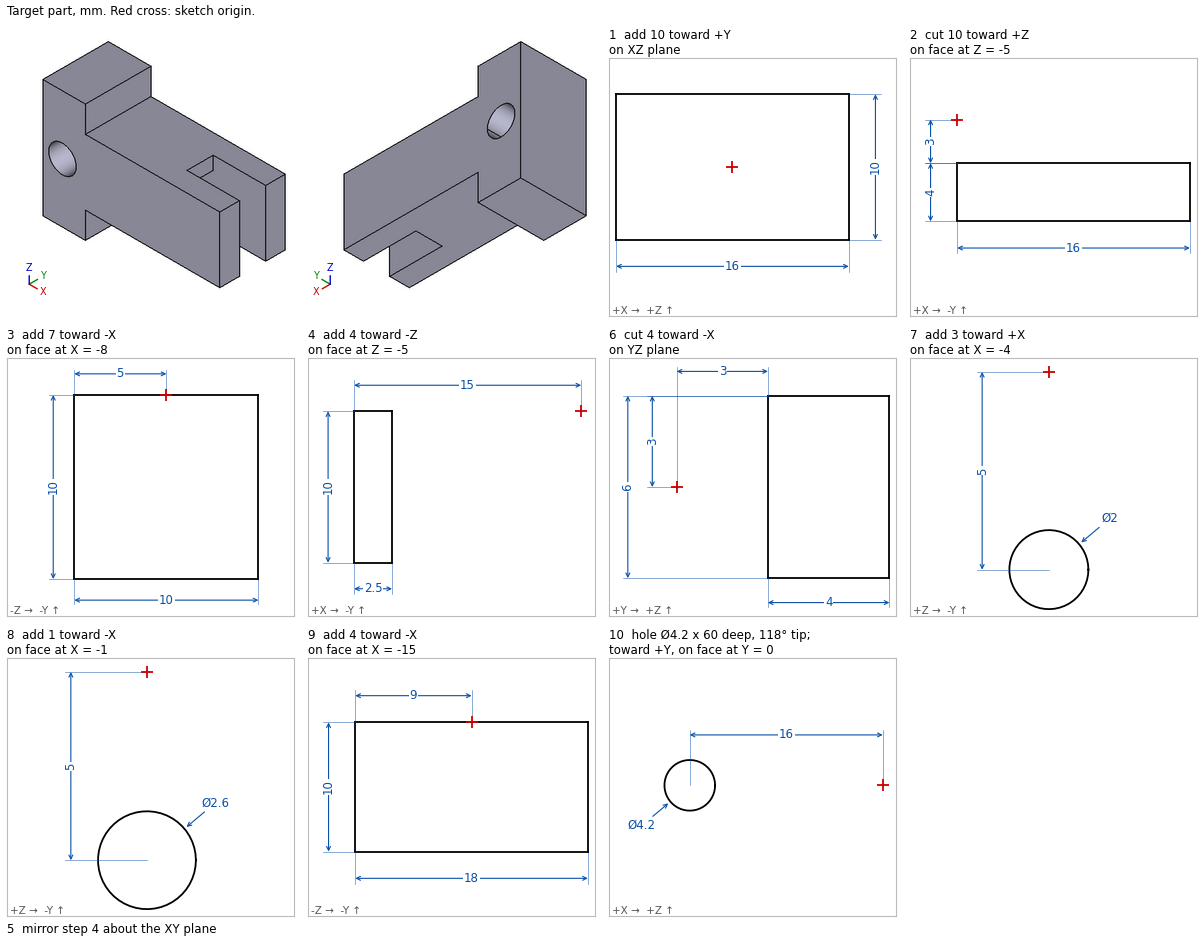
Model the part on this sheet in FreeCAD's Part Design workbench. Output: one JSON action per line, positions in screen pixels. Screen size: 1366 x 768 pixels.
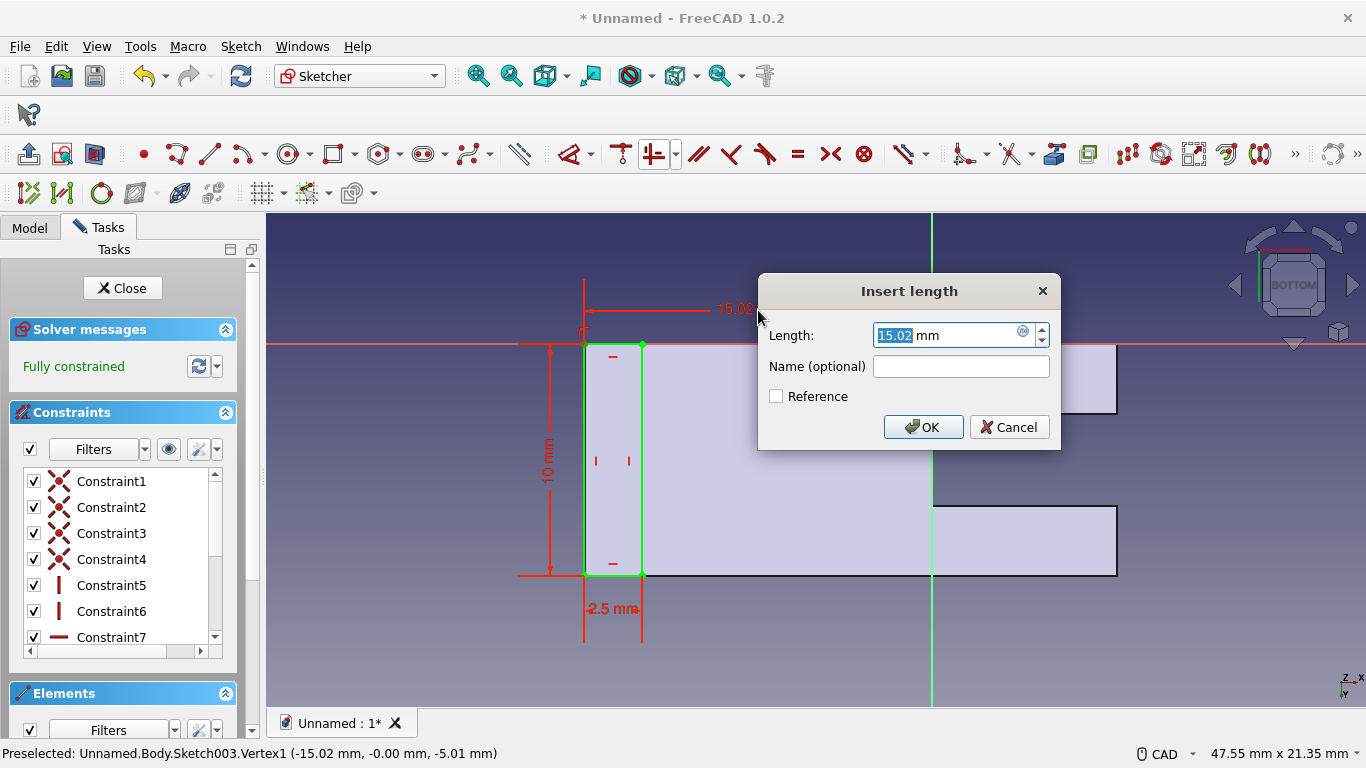
{"action": "type", "text": "15"}
{"action": "key", "text": "Return"}
{"action": "key", "text": "Escape"}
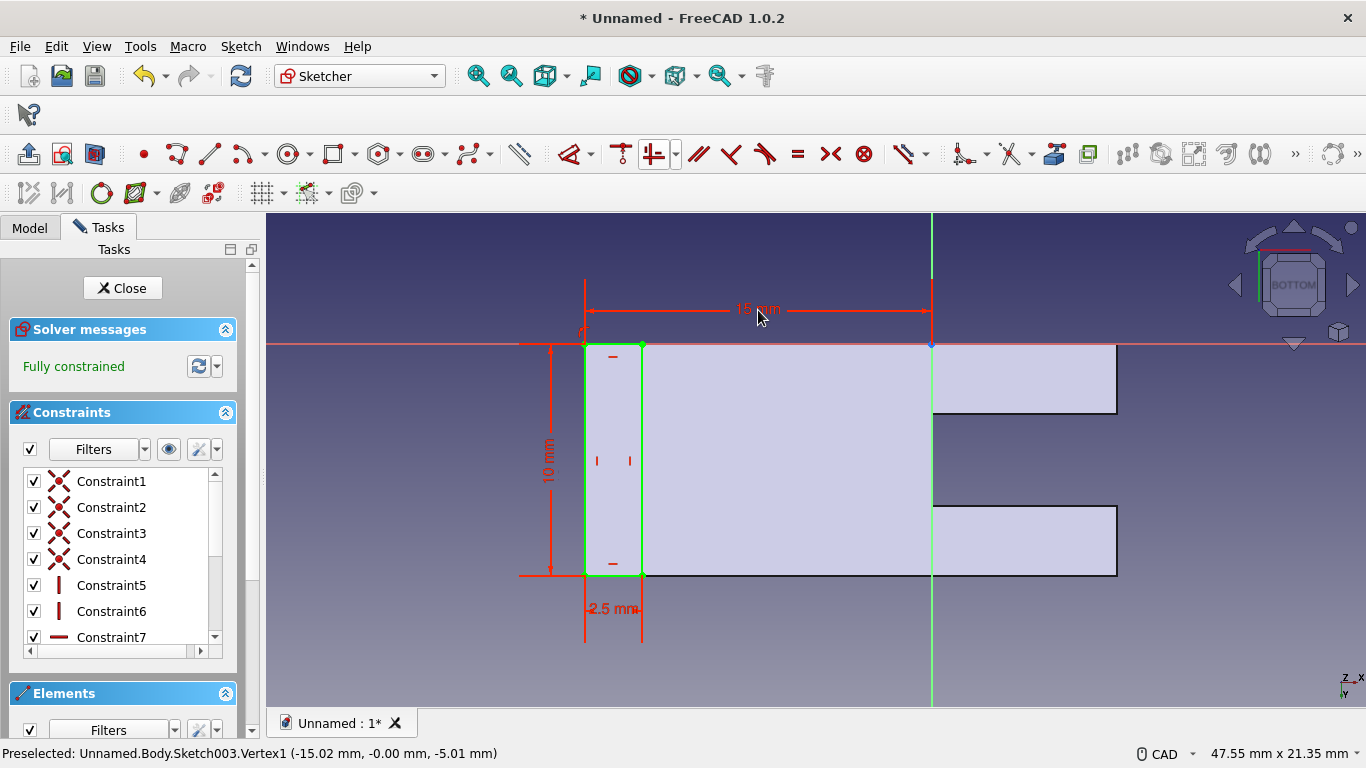
{"action": "left_click", "coordinate": [123, 288]}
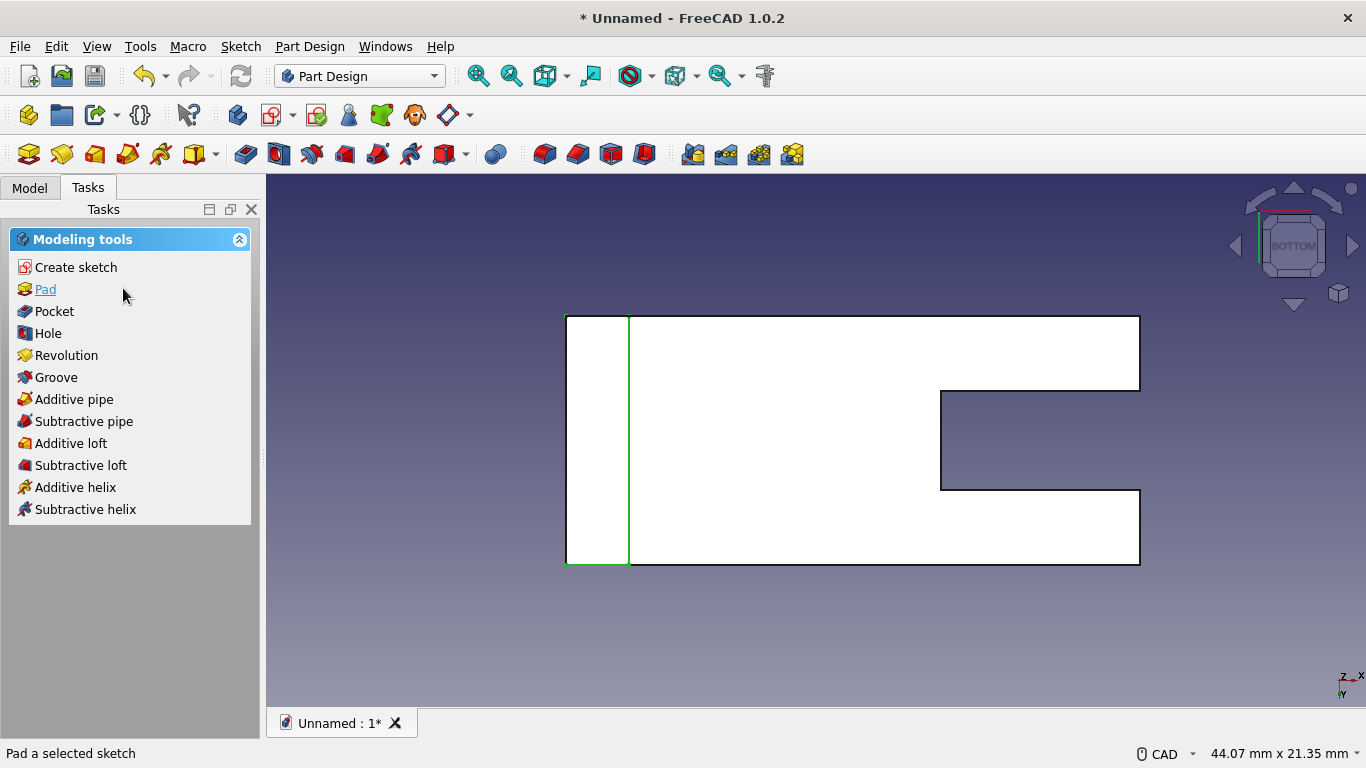
{"action": "left_click", "coordinate": [29, 154]}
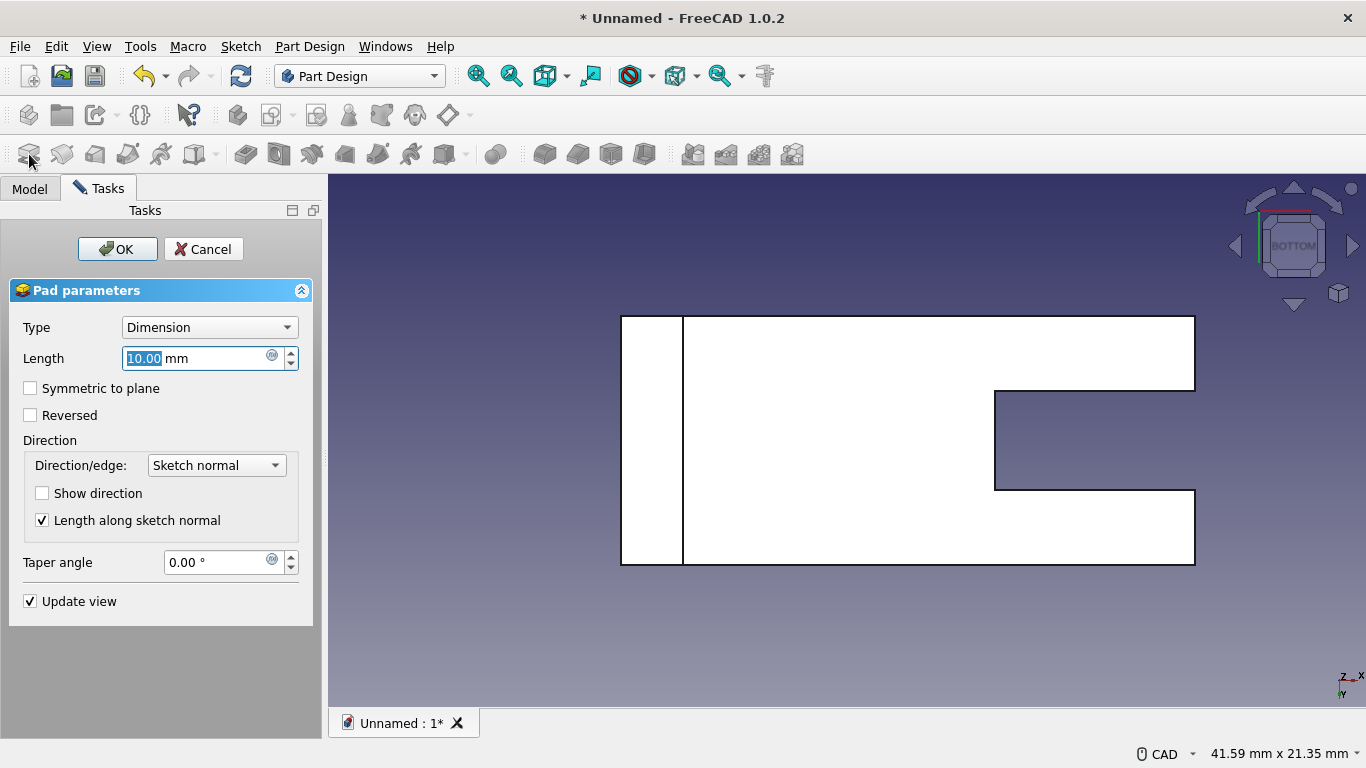
{"action": "type", "text": "4"}
{"action": "key", "text": "Tab"}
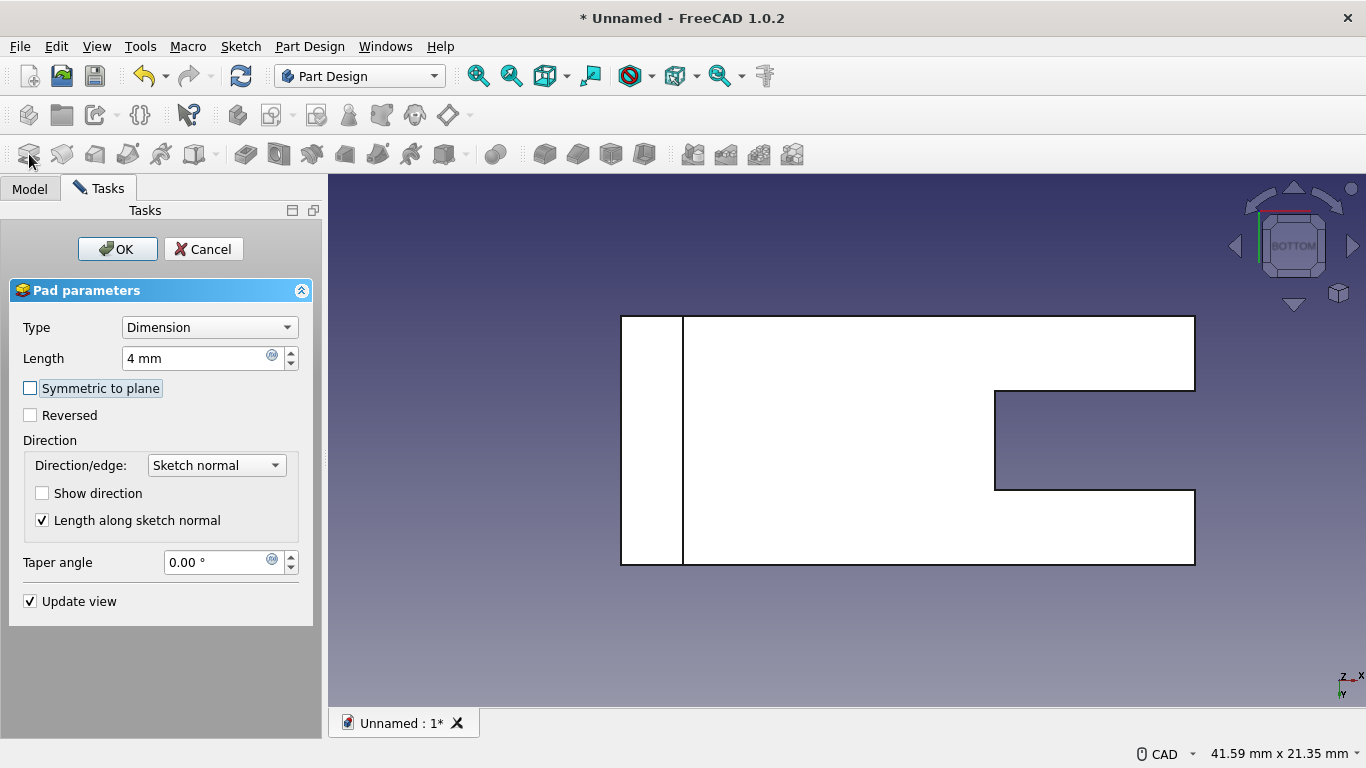
{"action": "left_click", "coordinate": [118, 249]}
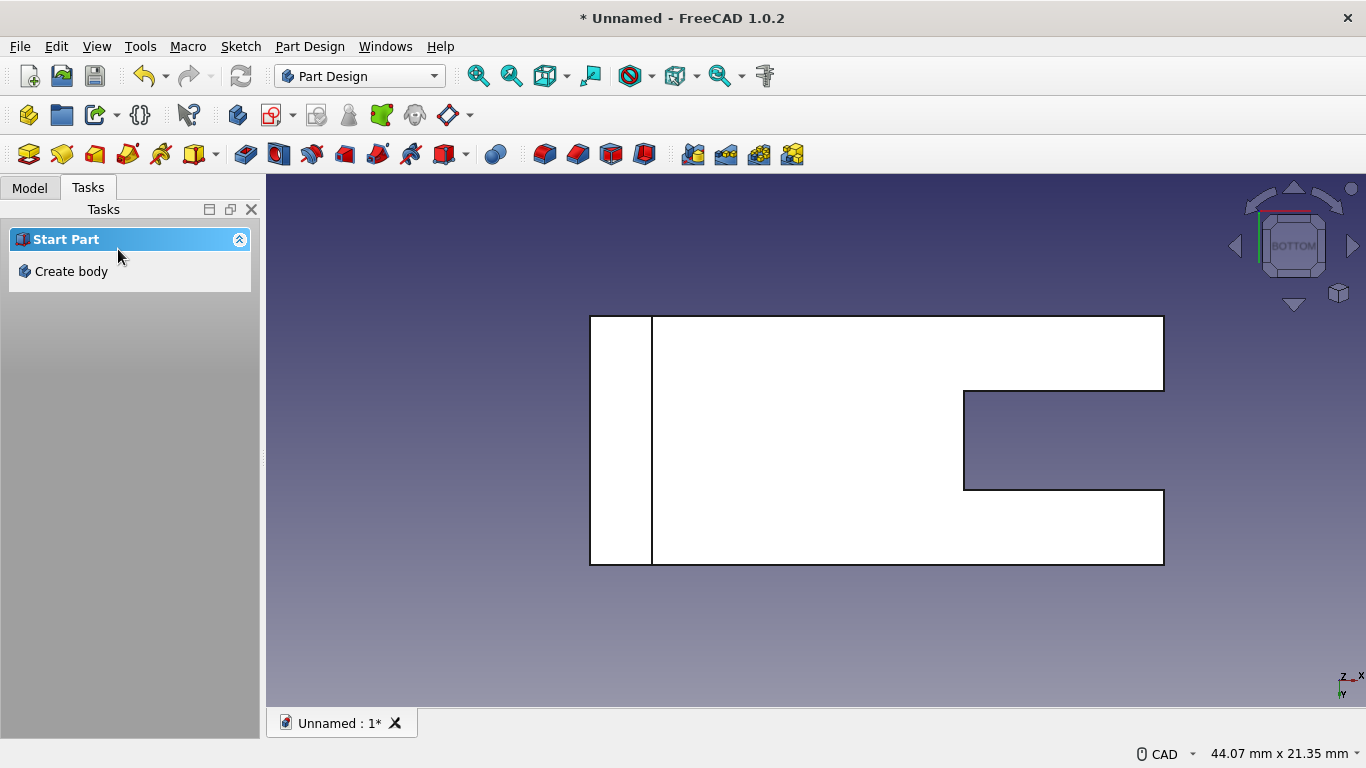
{"action": "left_click", "coordinate": [30, 188]}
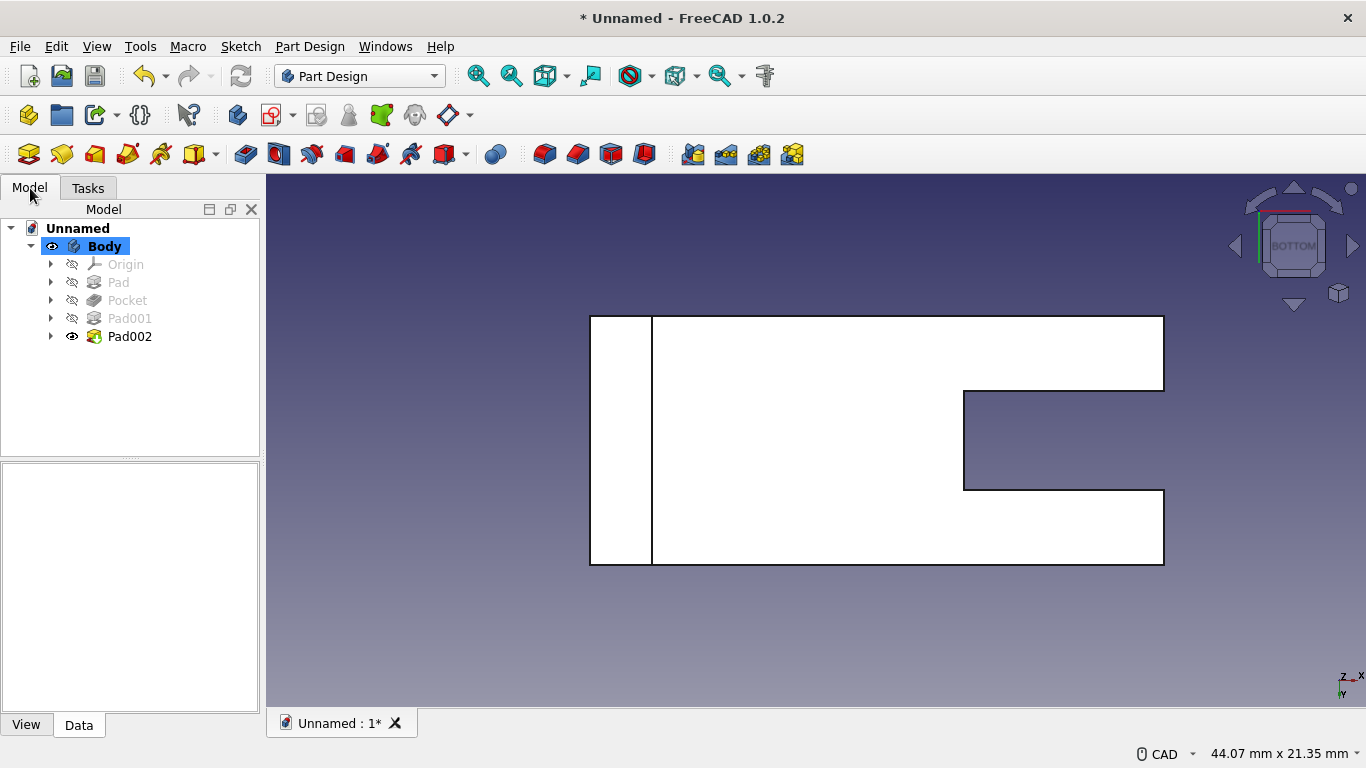
{"action": "left_click", "coordinate": [117, 336]}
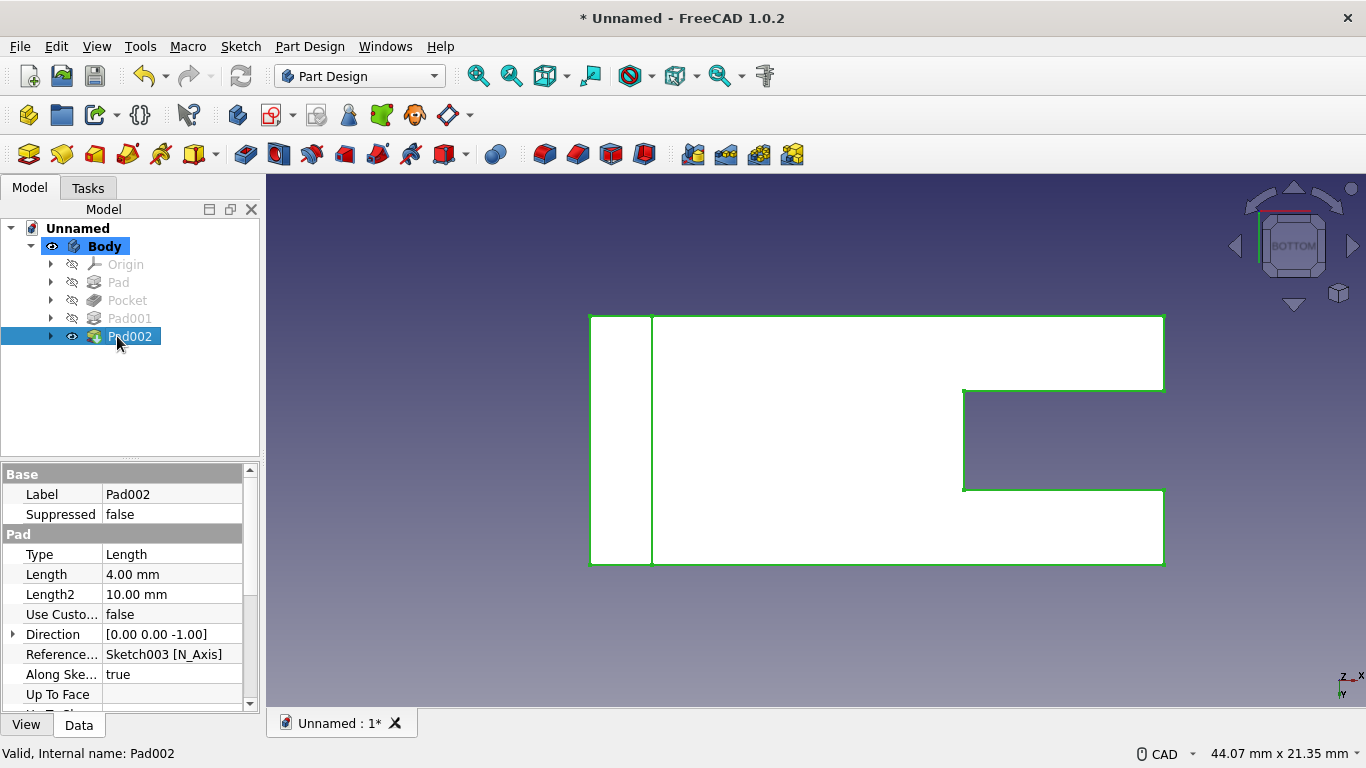
{"action": "left_click", "coordinate": [693, 154]}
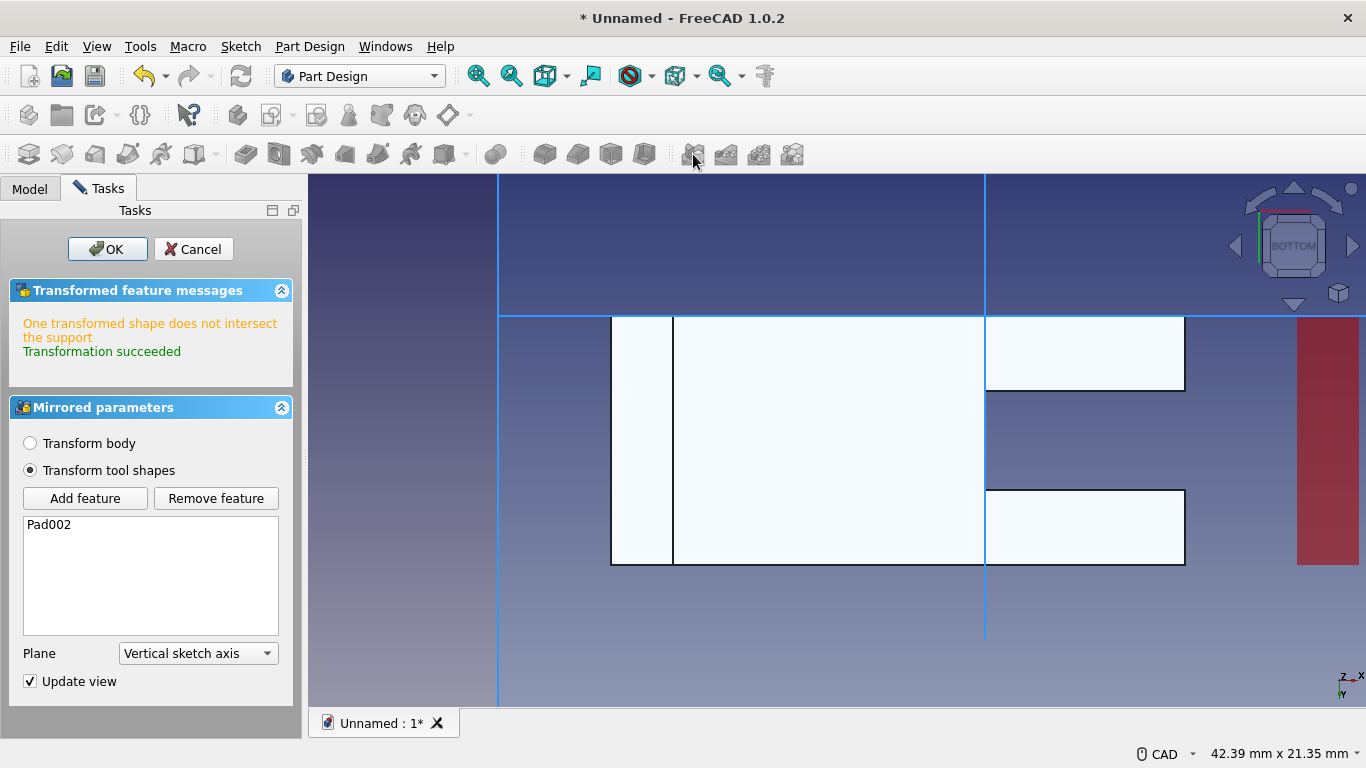
{"action": "left_click", "coordinate": [199, 654]}